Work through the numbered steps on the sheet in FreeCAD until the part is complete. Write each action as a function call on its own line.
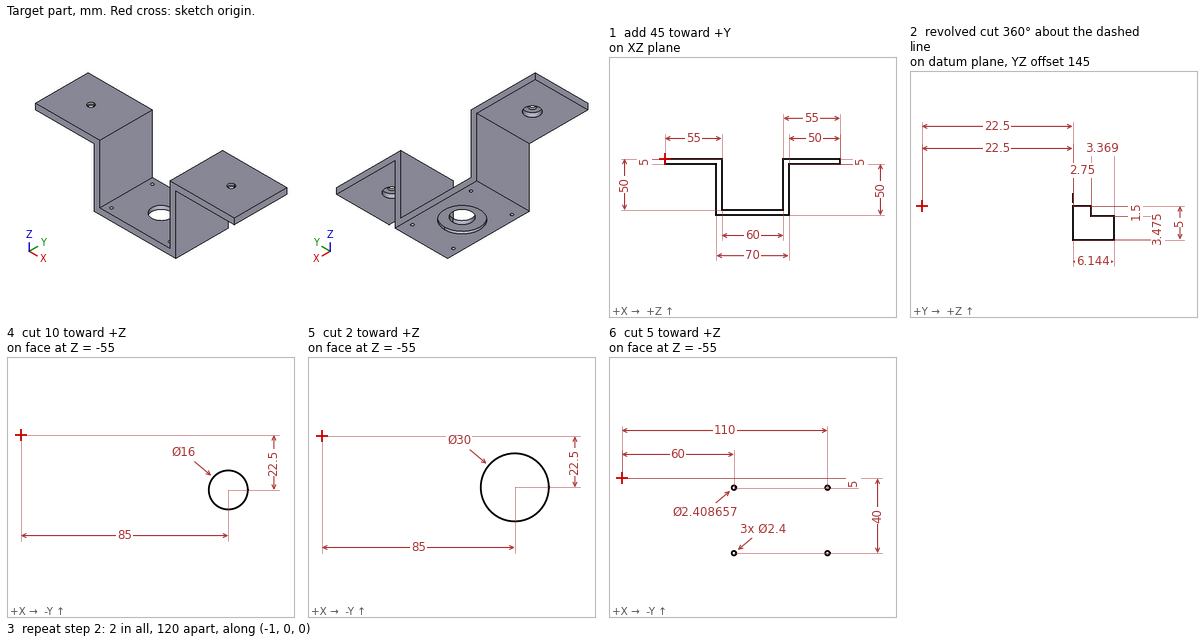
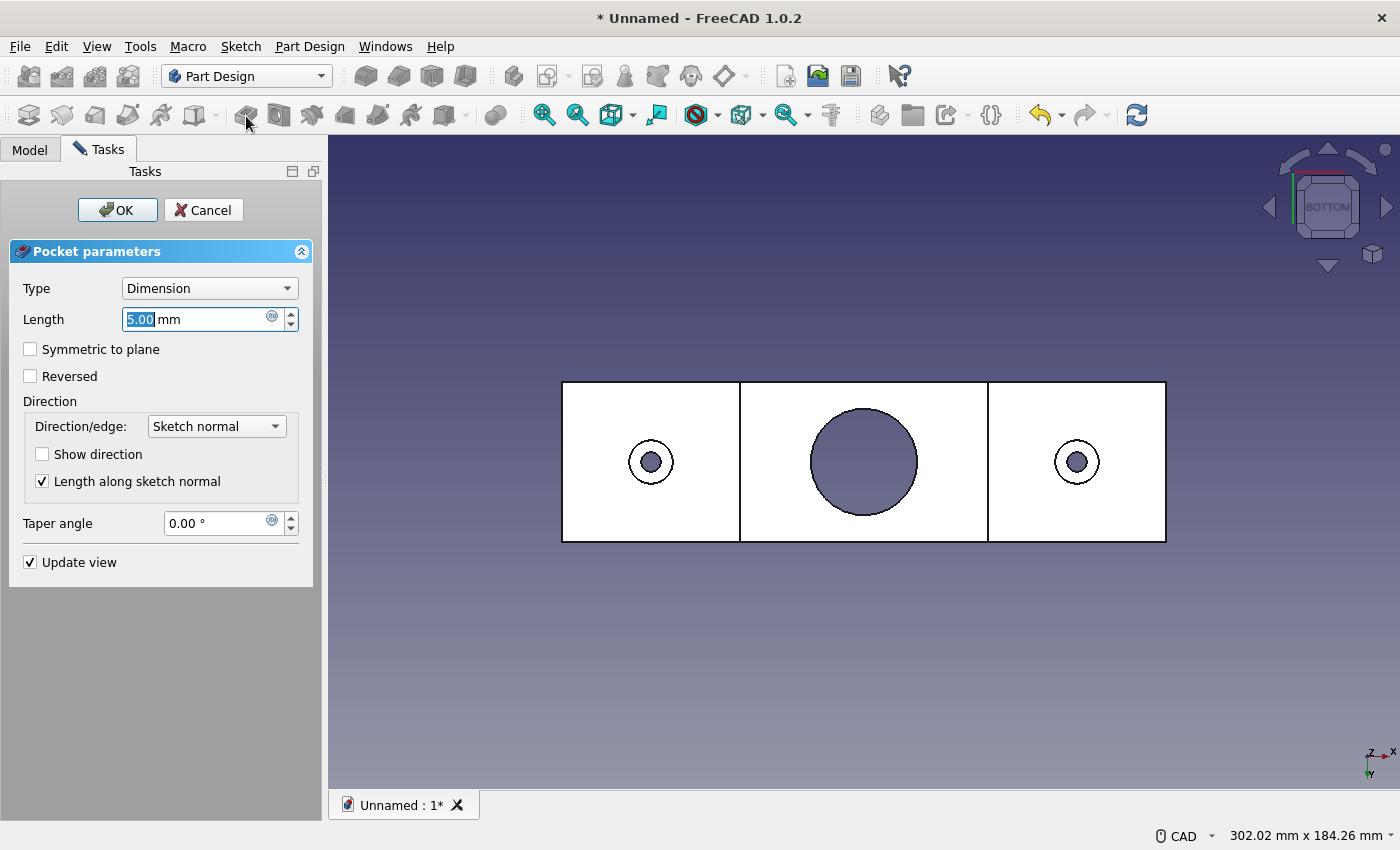
text(2)
key(Tab)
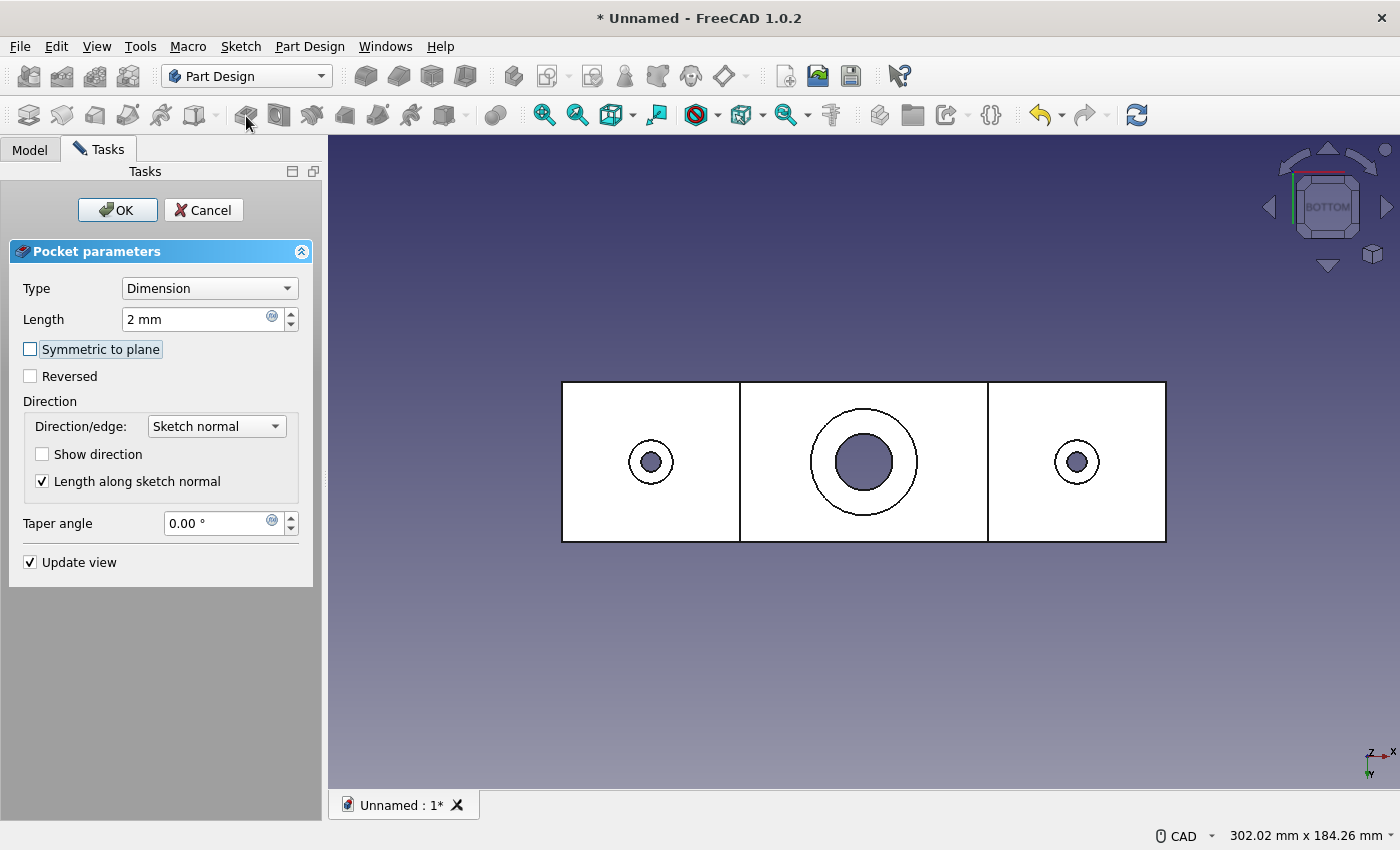
click(118, 210)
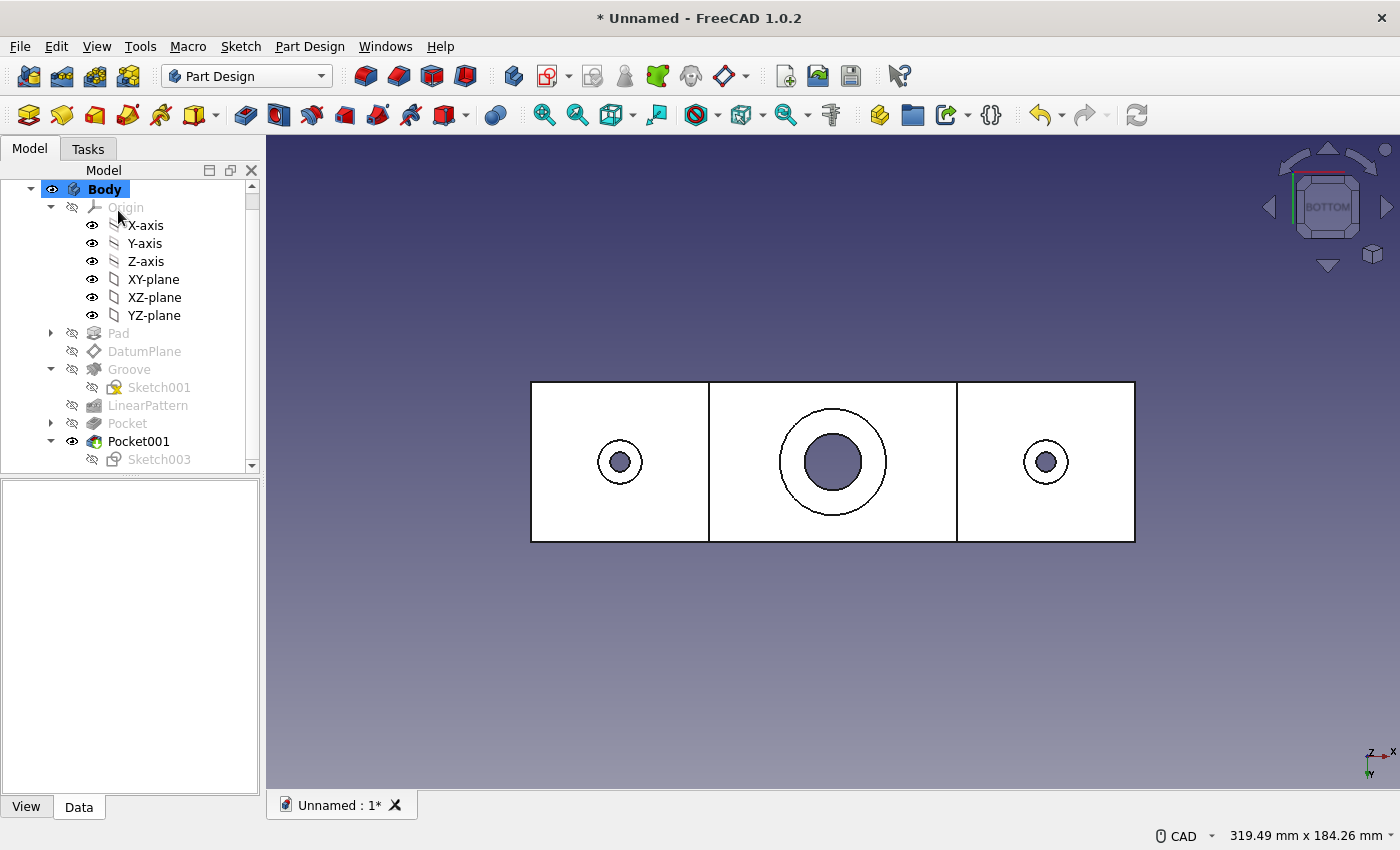
click(904, 507)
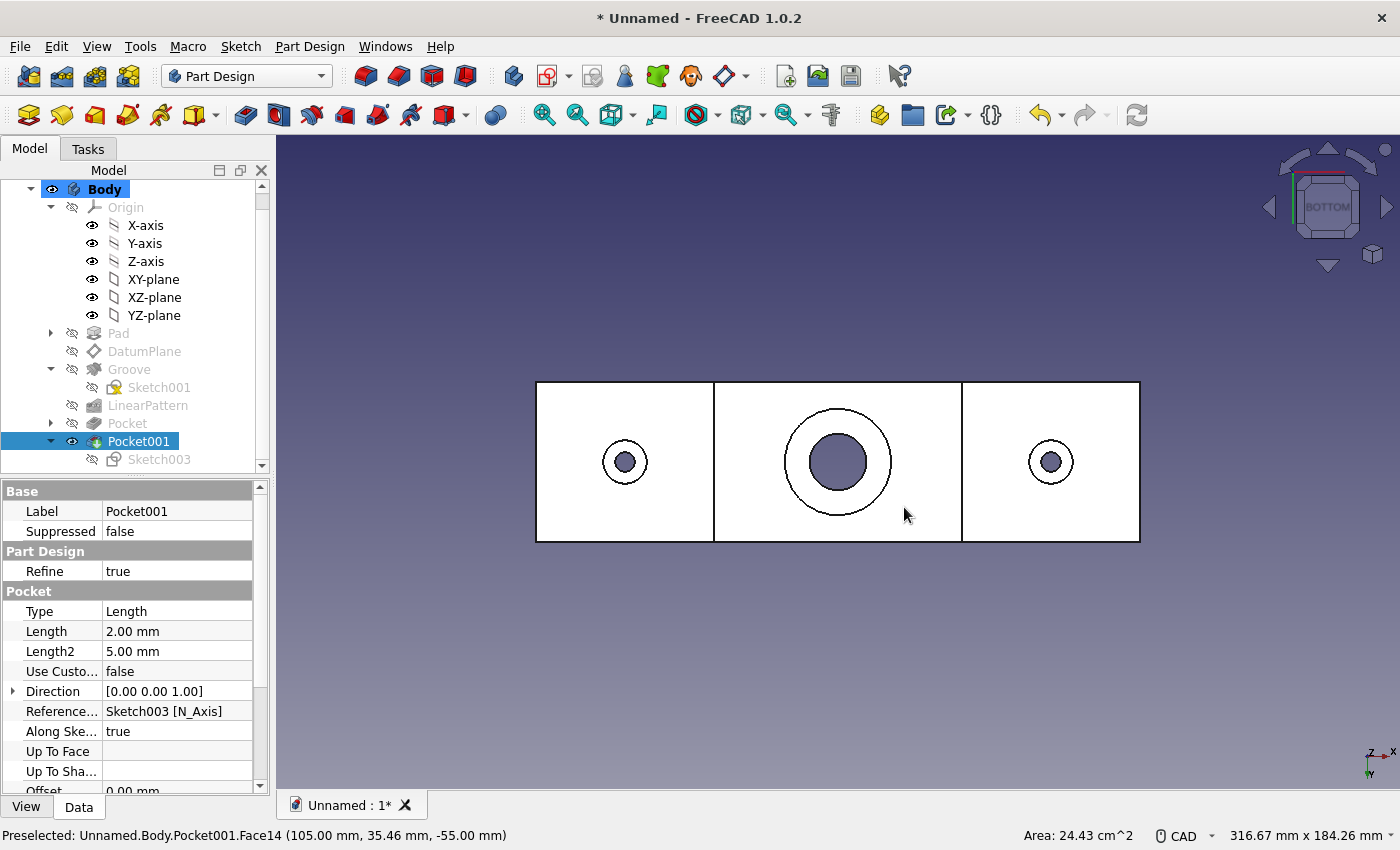
click(546, 76)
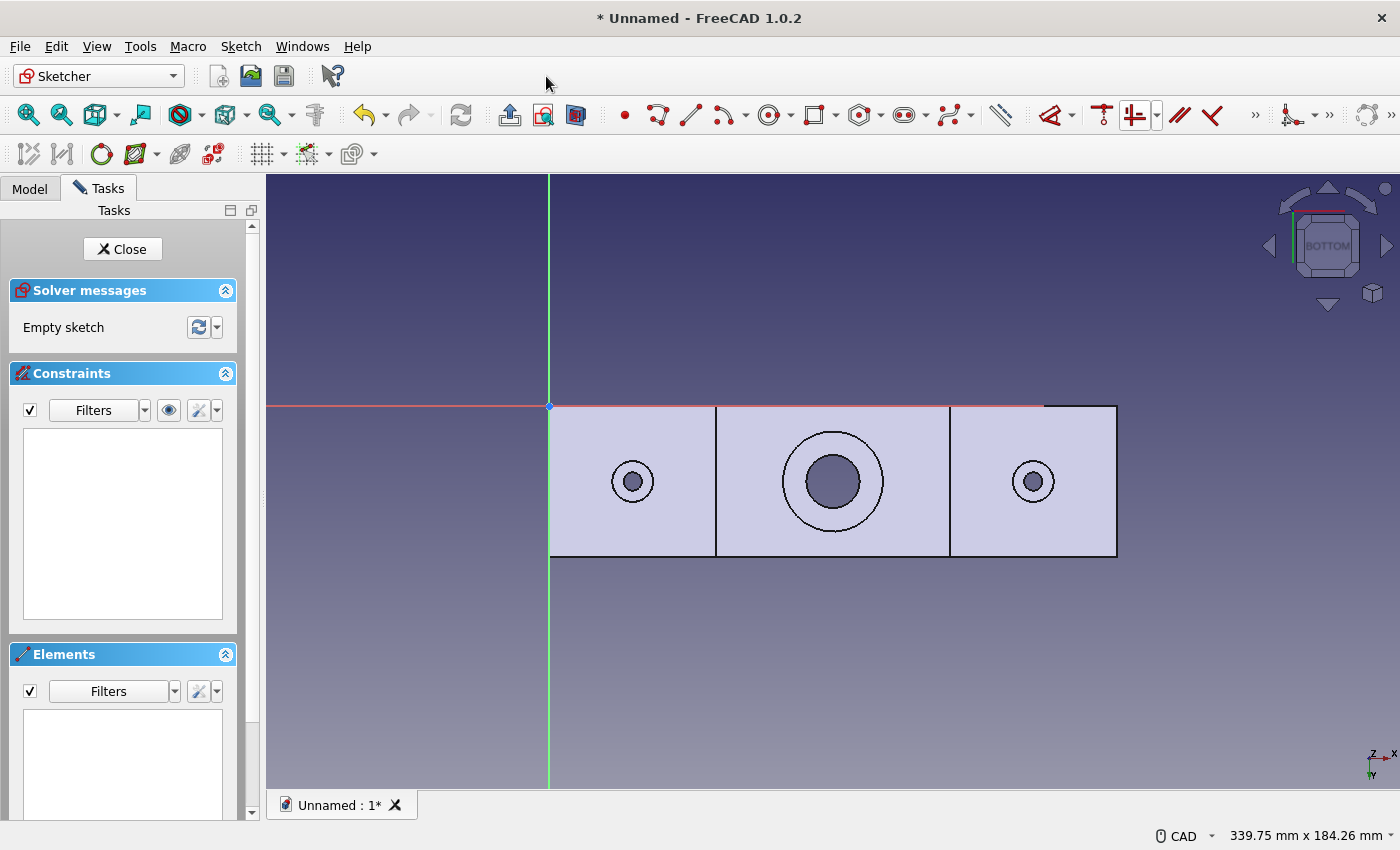
scroll(699, 467, up, 3)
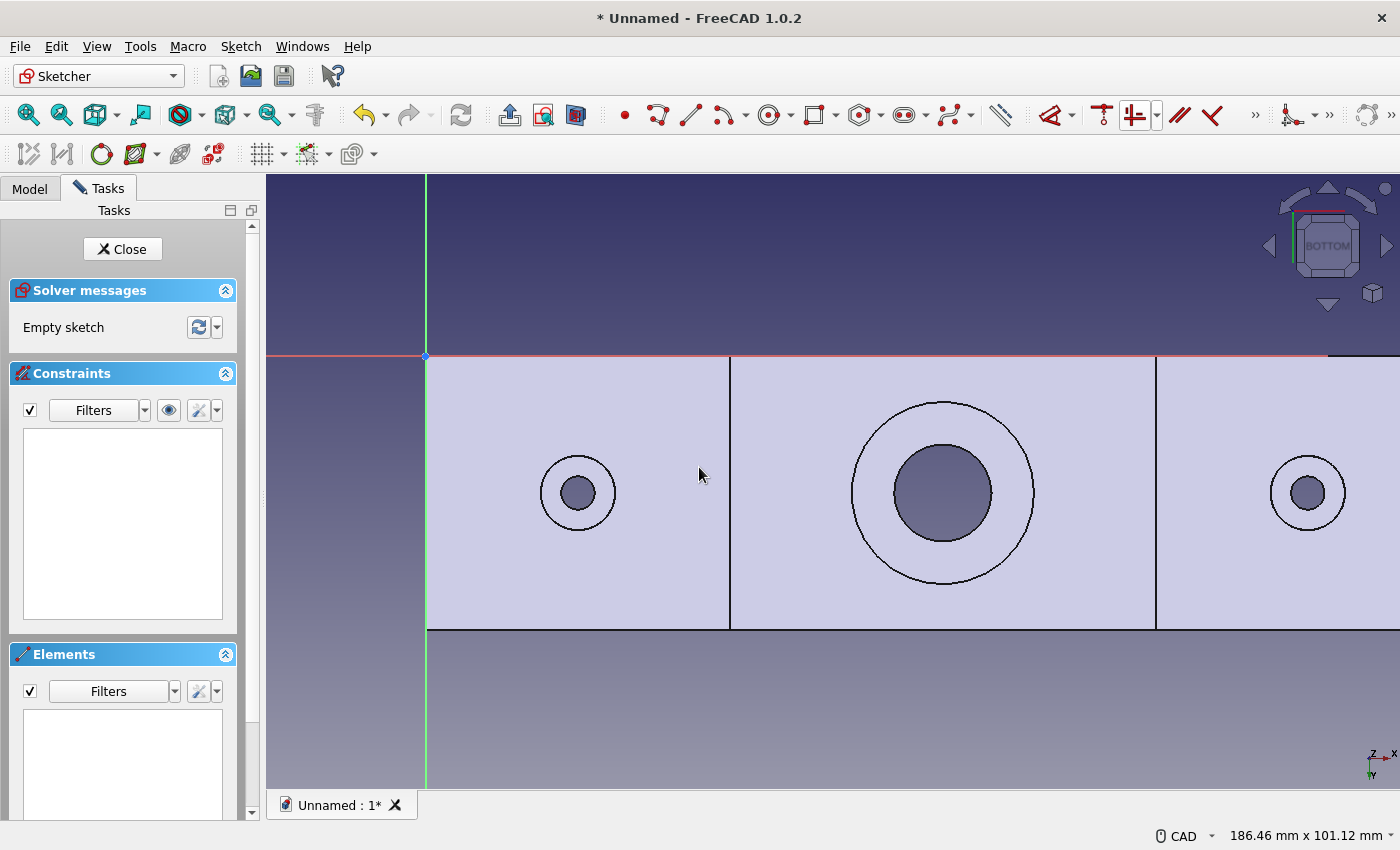
click(768, 116)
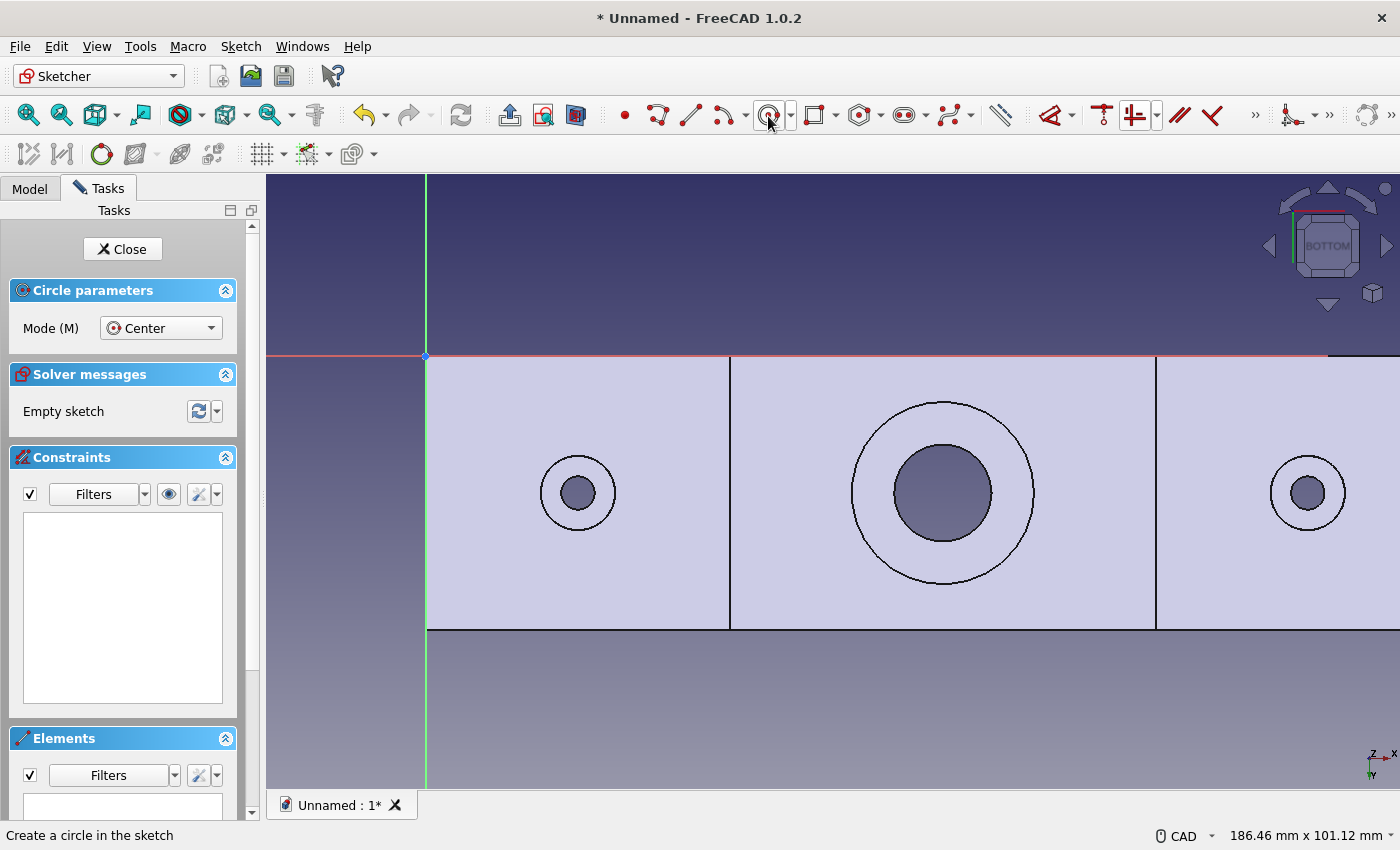
scroll(791, 387, up, 6)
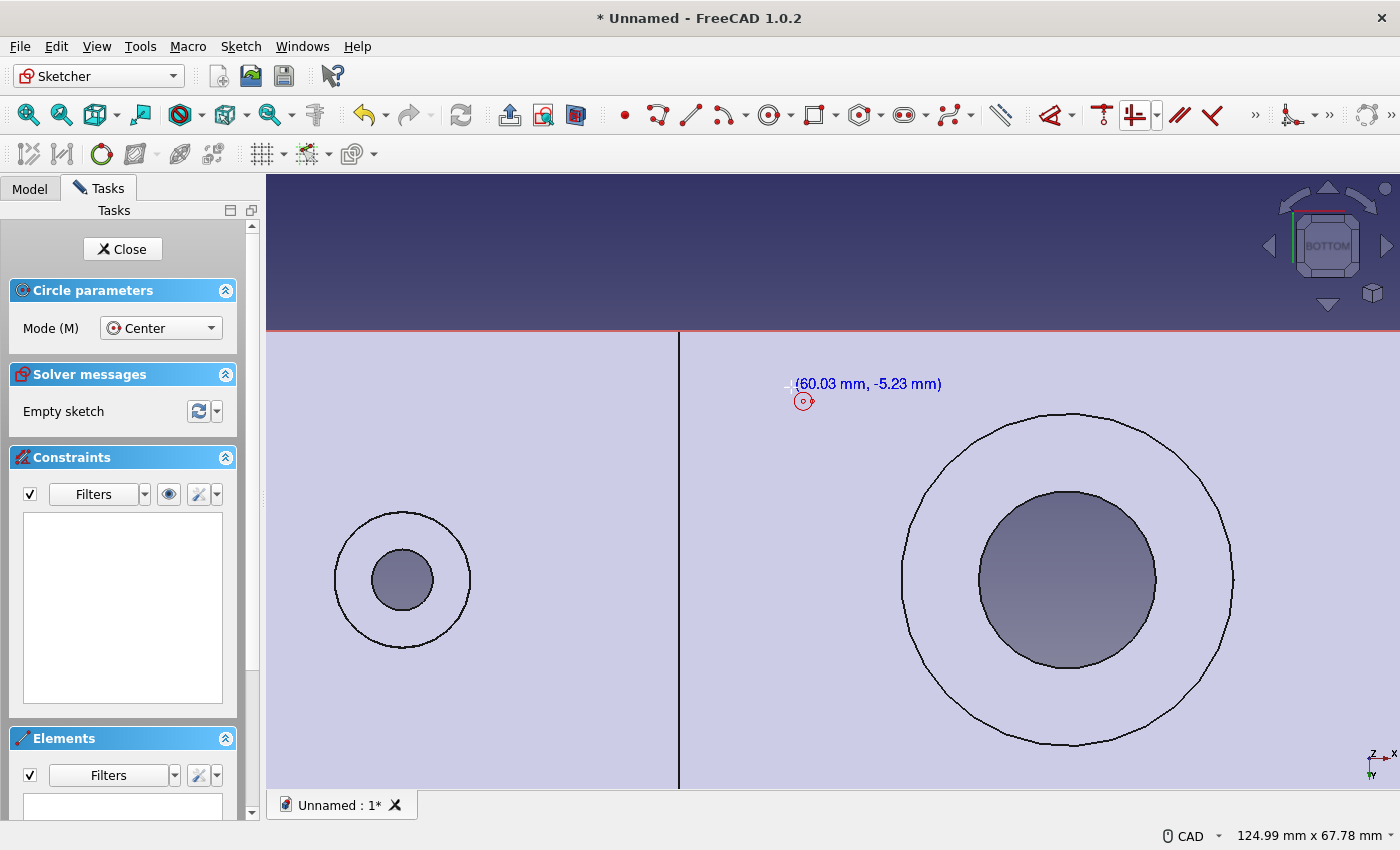
click(789, 385)
click(806, 368)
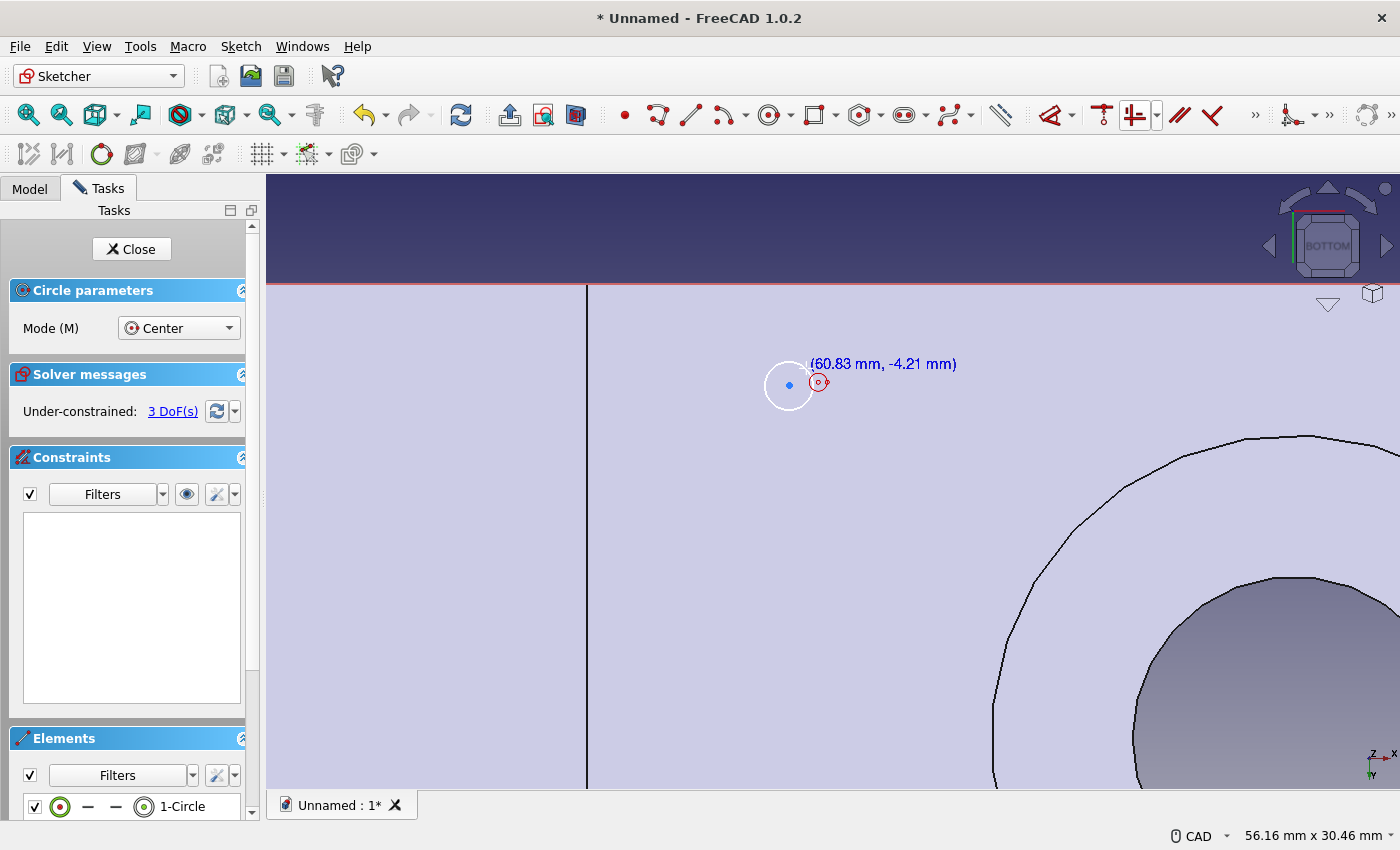
scroll(792, 387, down, 6)